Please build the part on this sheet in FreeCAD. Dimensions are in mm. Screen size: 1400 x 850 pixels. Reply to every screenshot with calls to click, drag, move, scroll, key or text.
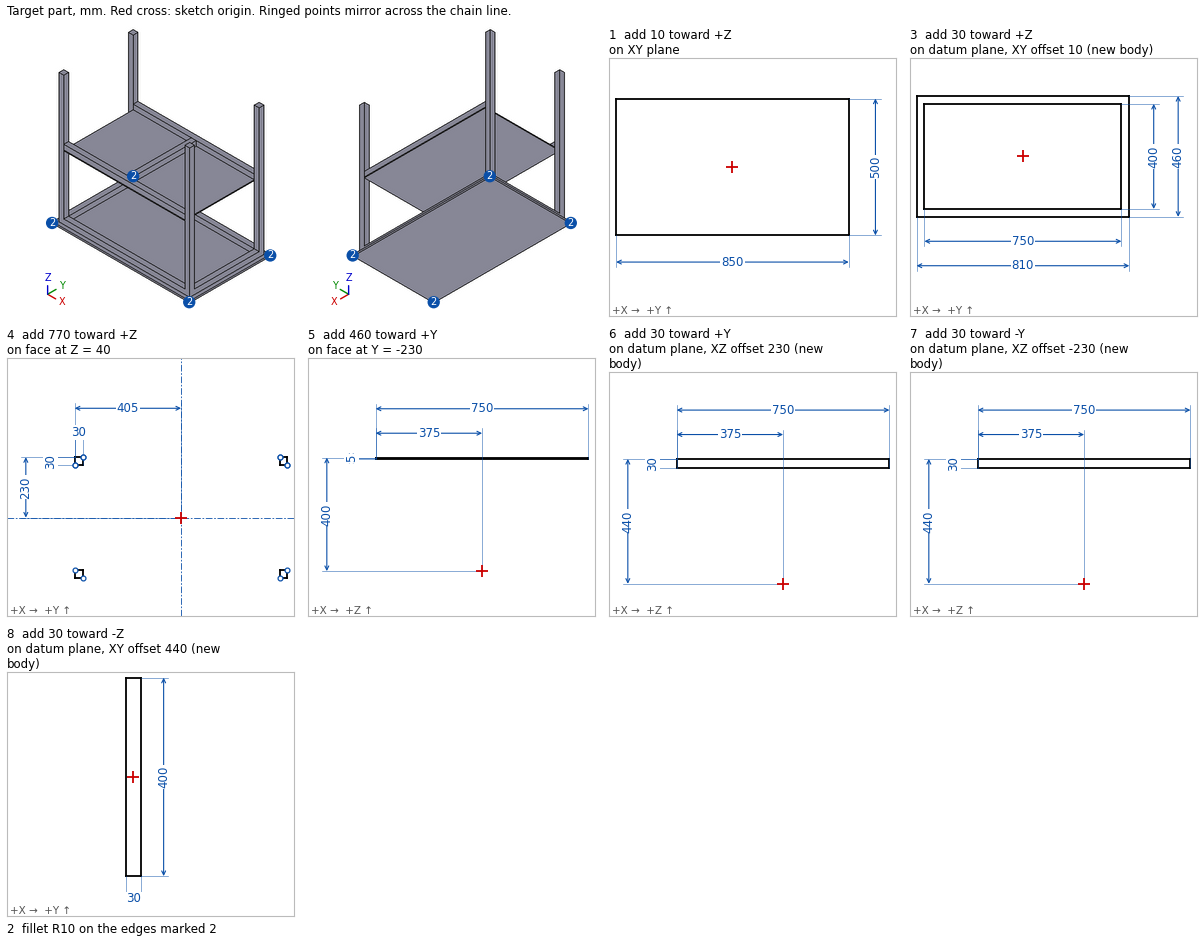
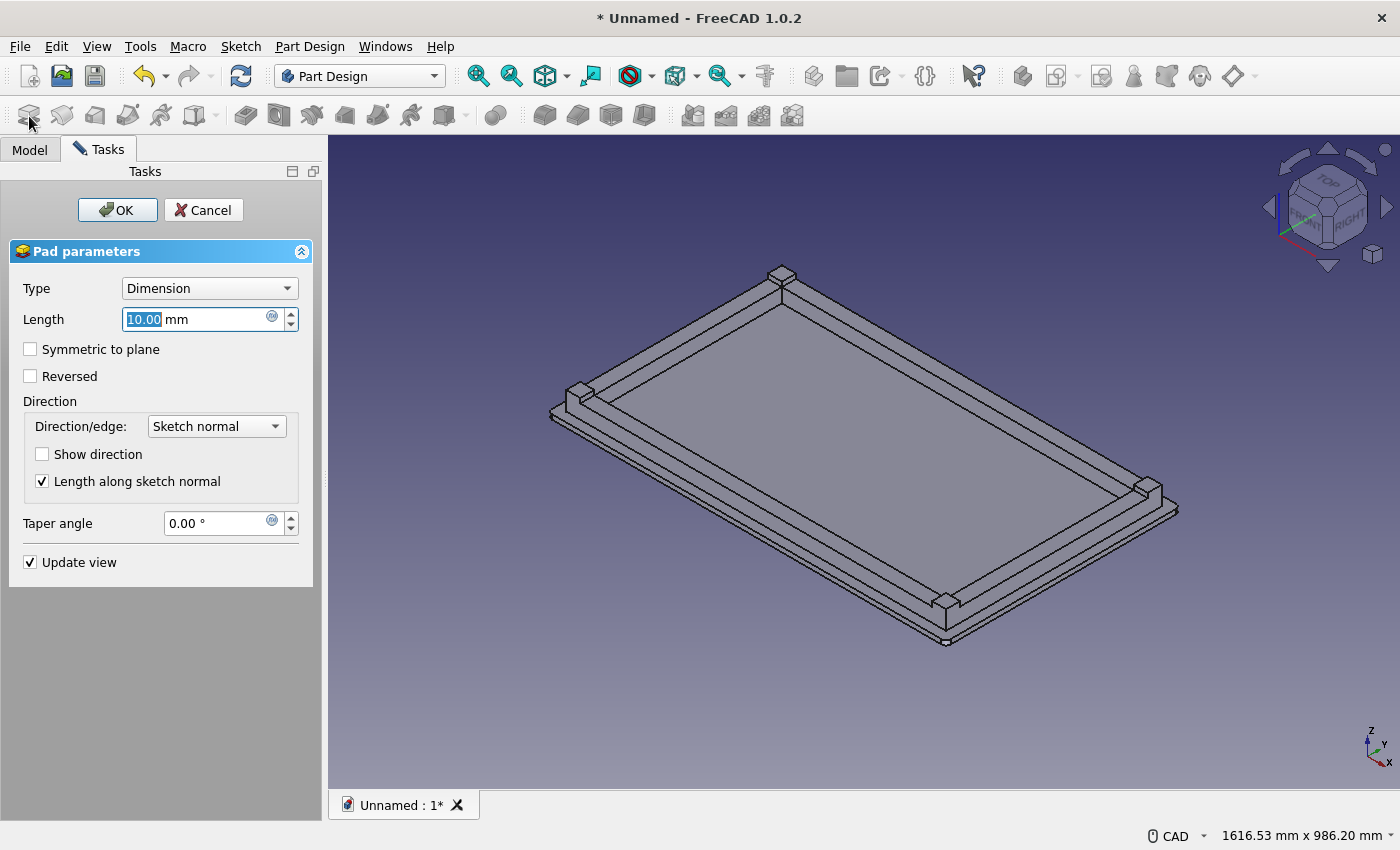
text(770)
key(Tab)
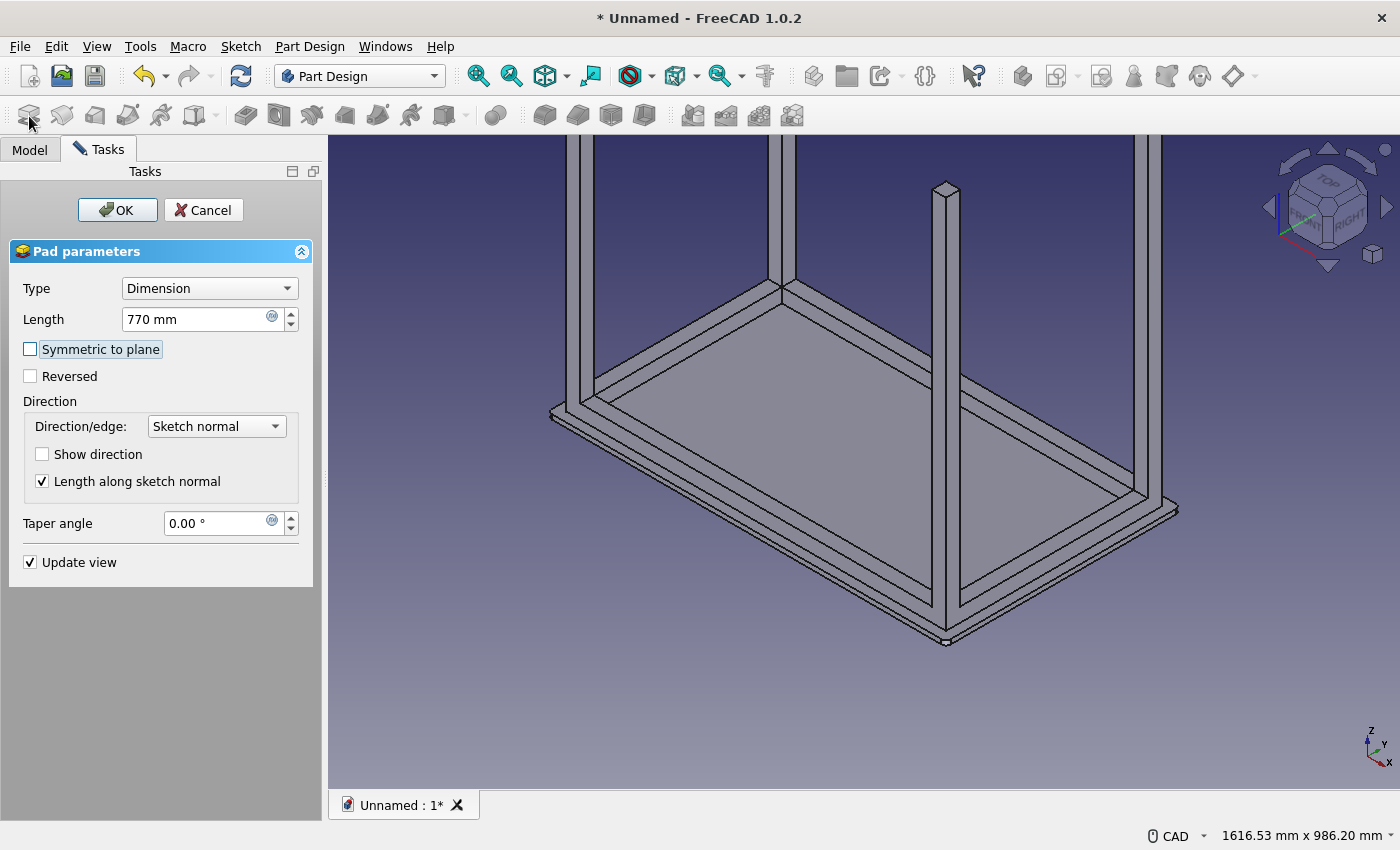
click(118, 210)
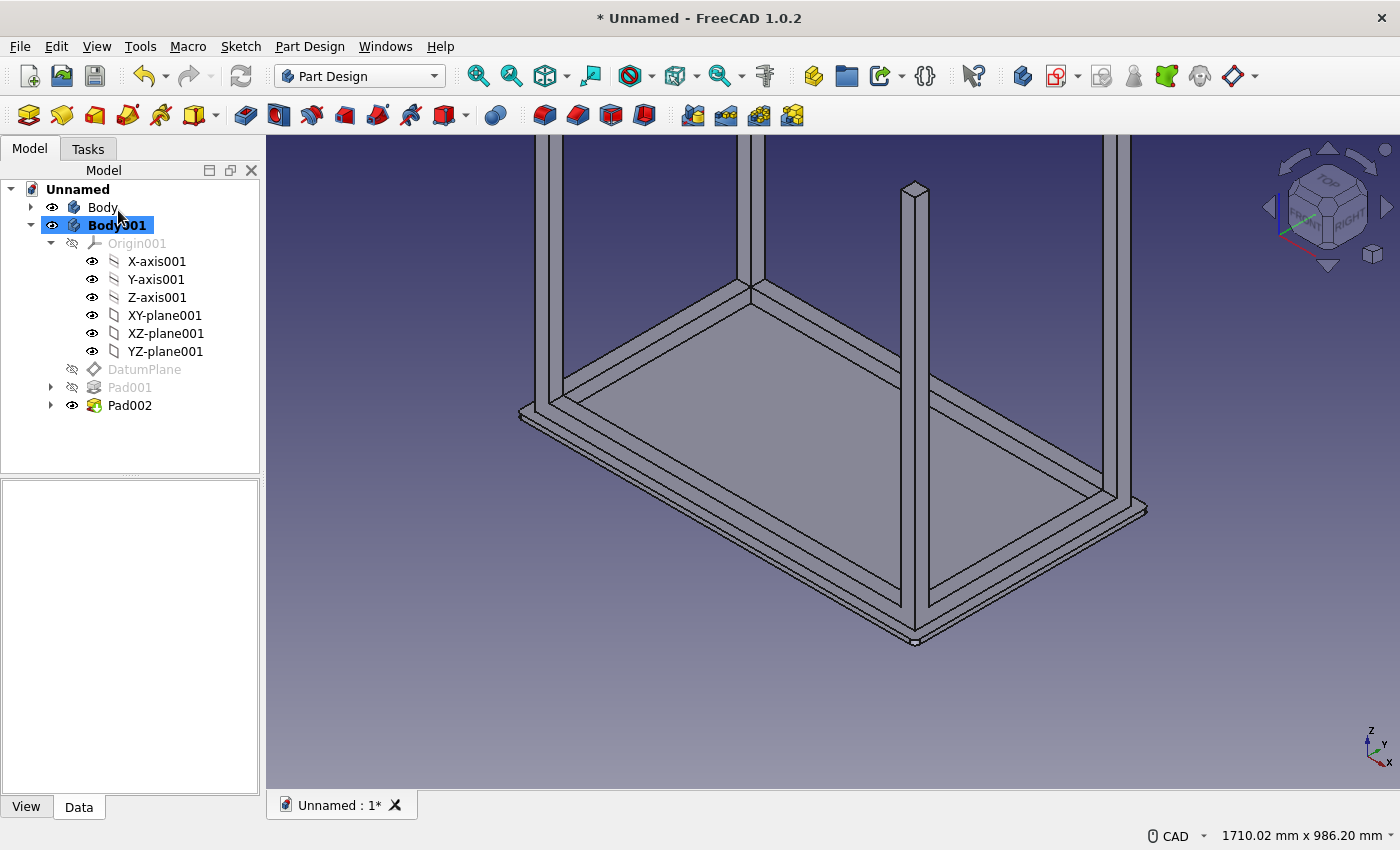
click(479, 76)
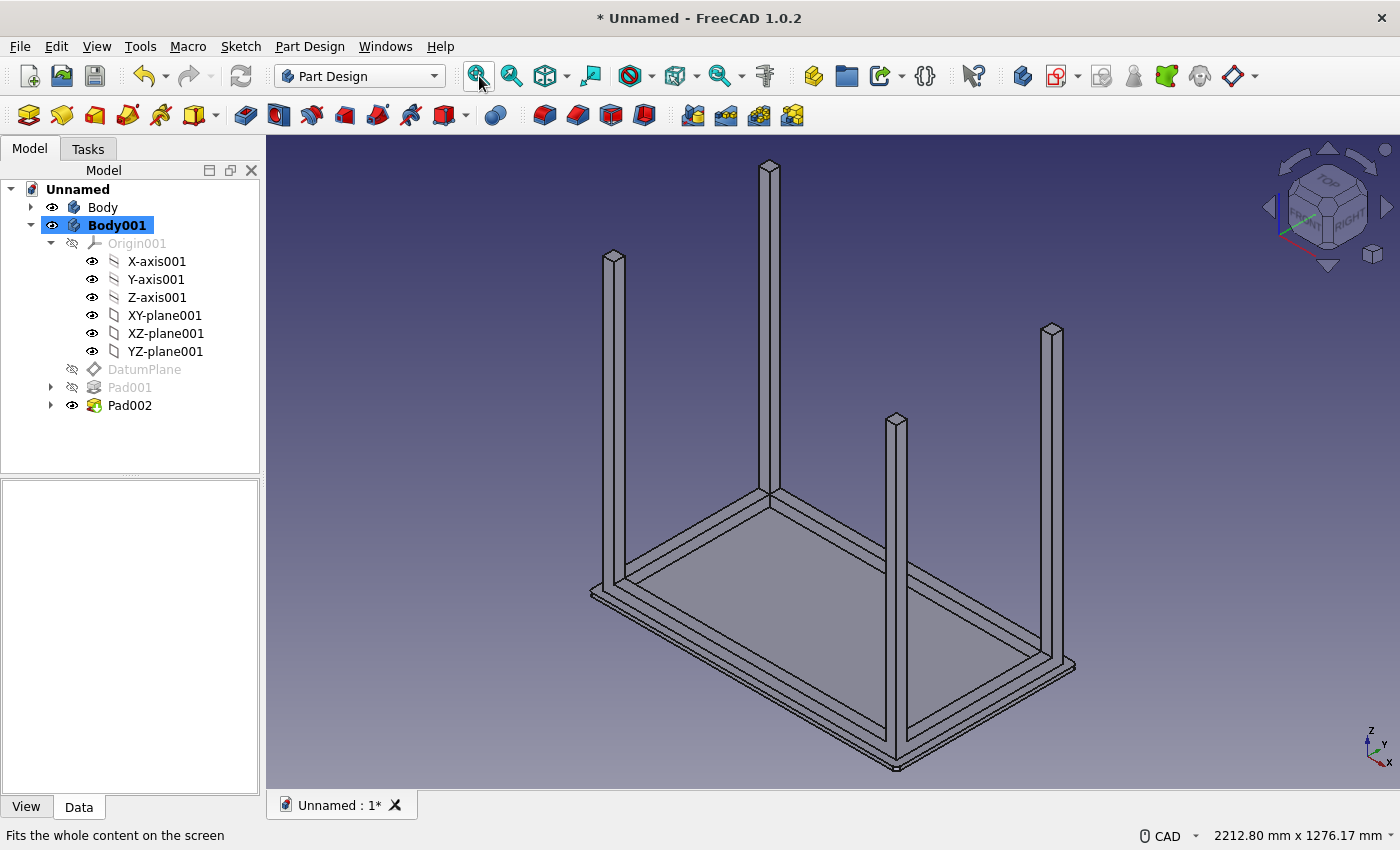
scroll(893, 641, up, 5)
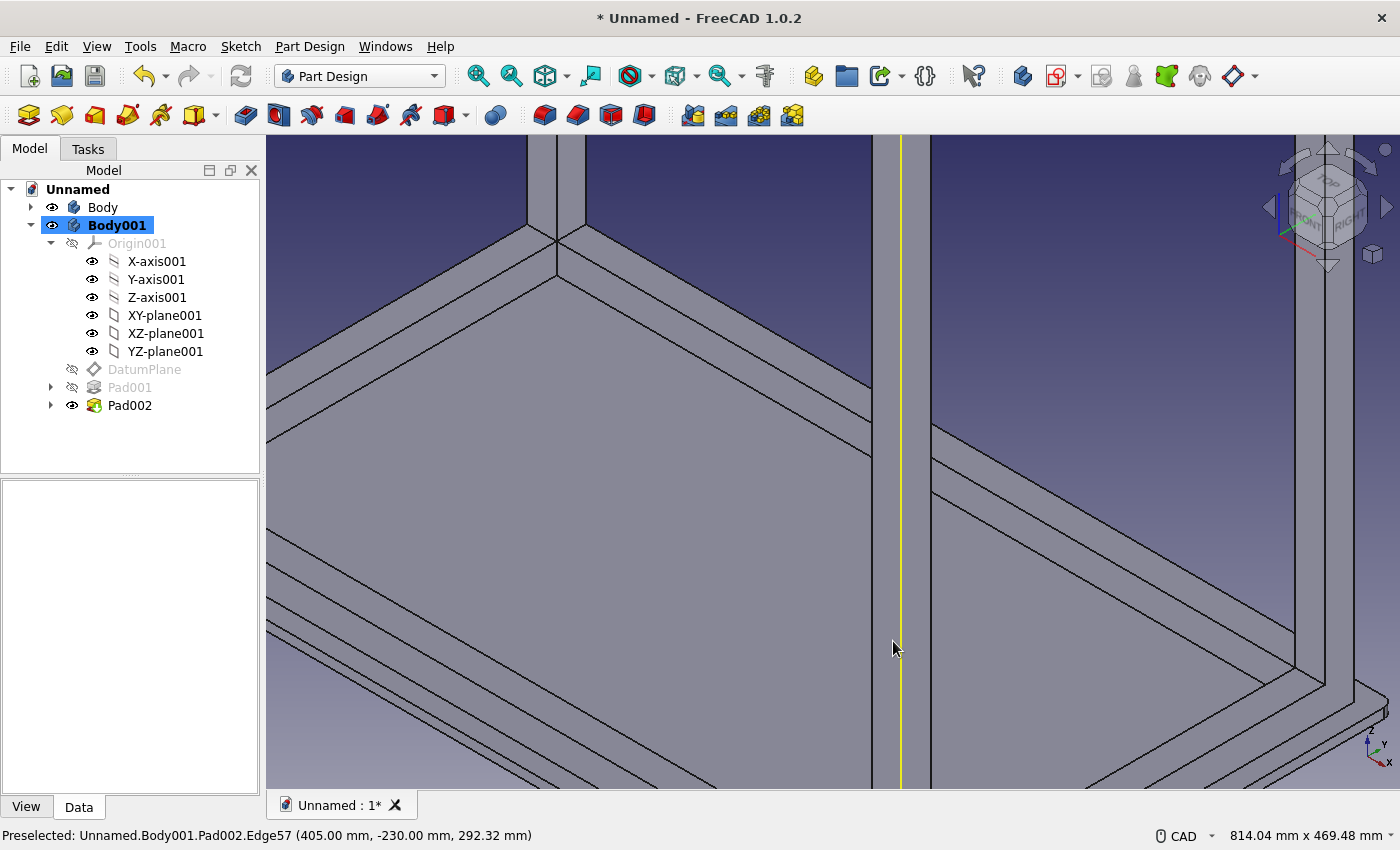
click(891, 642)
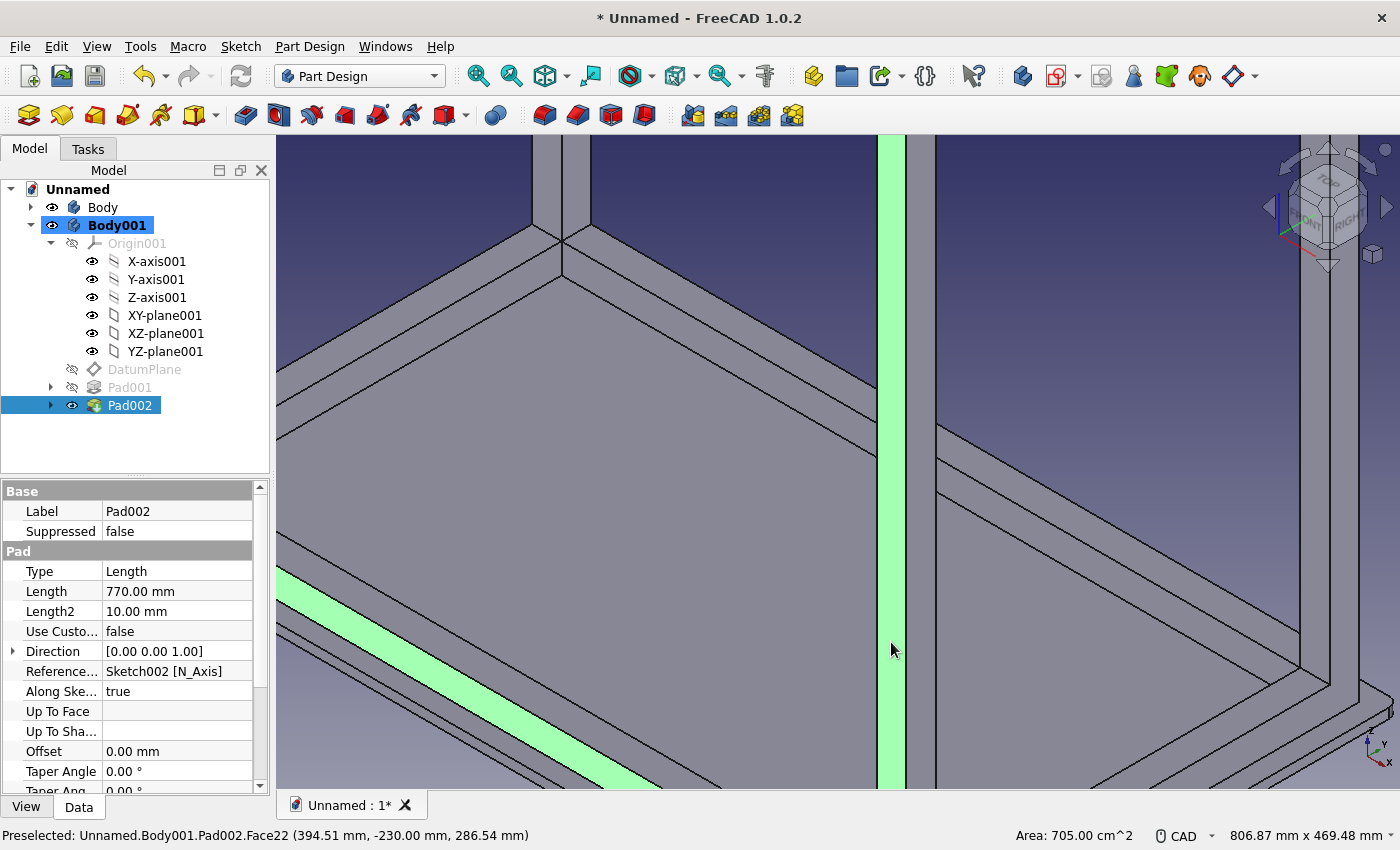
click(1056, 76)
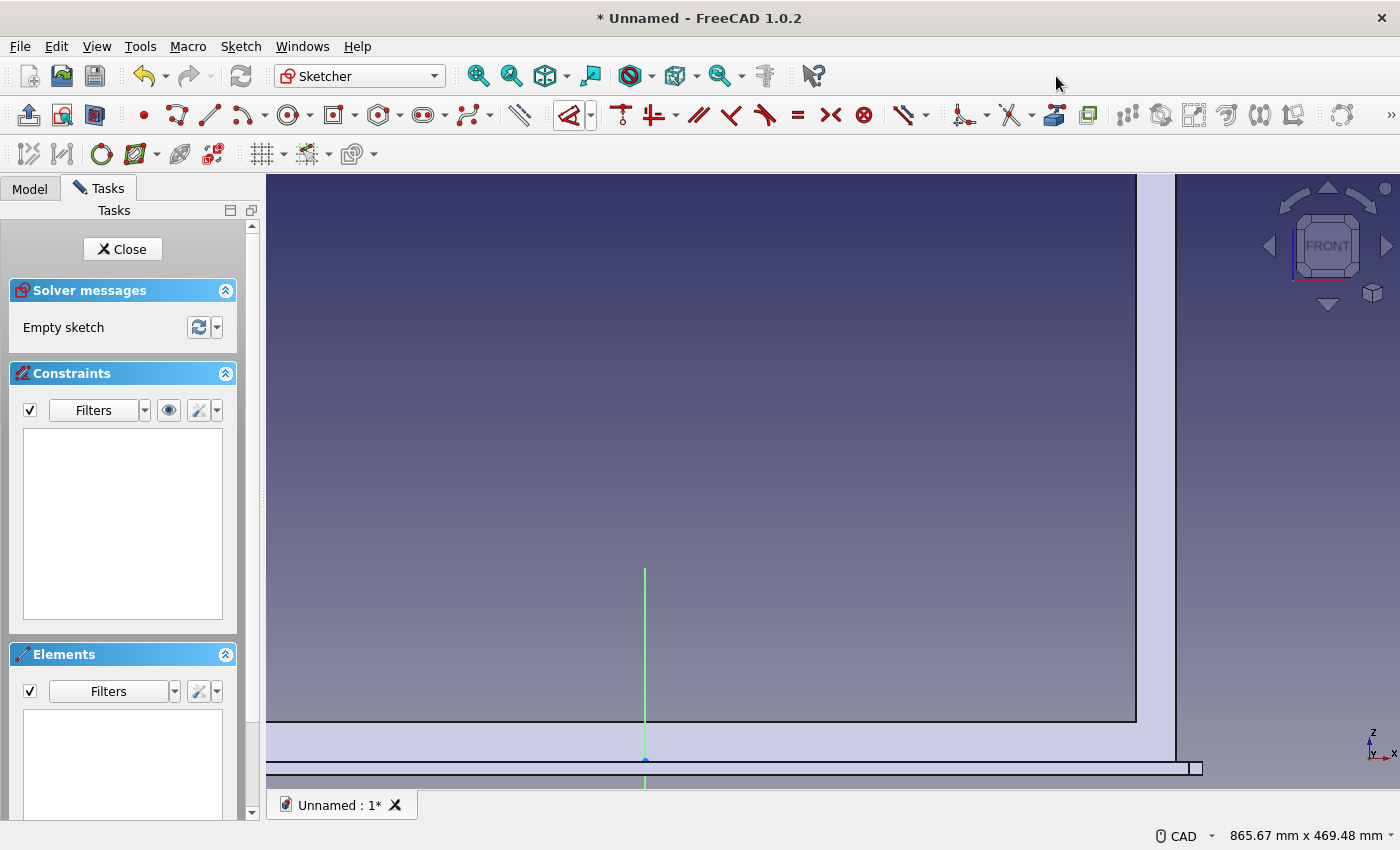
scroll(1007, 444, down, 2)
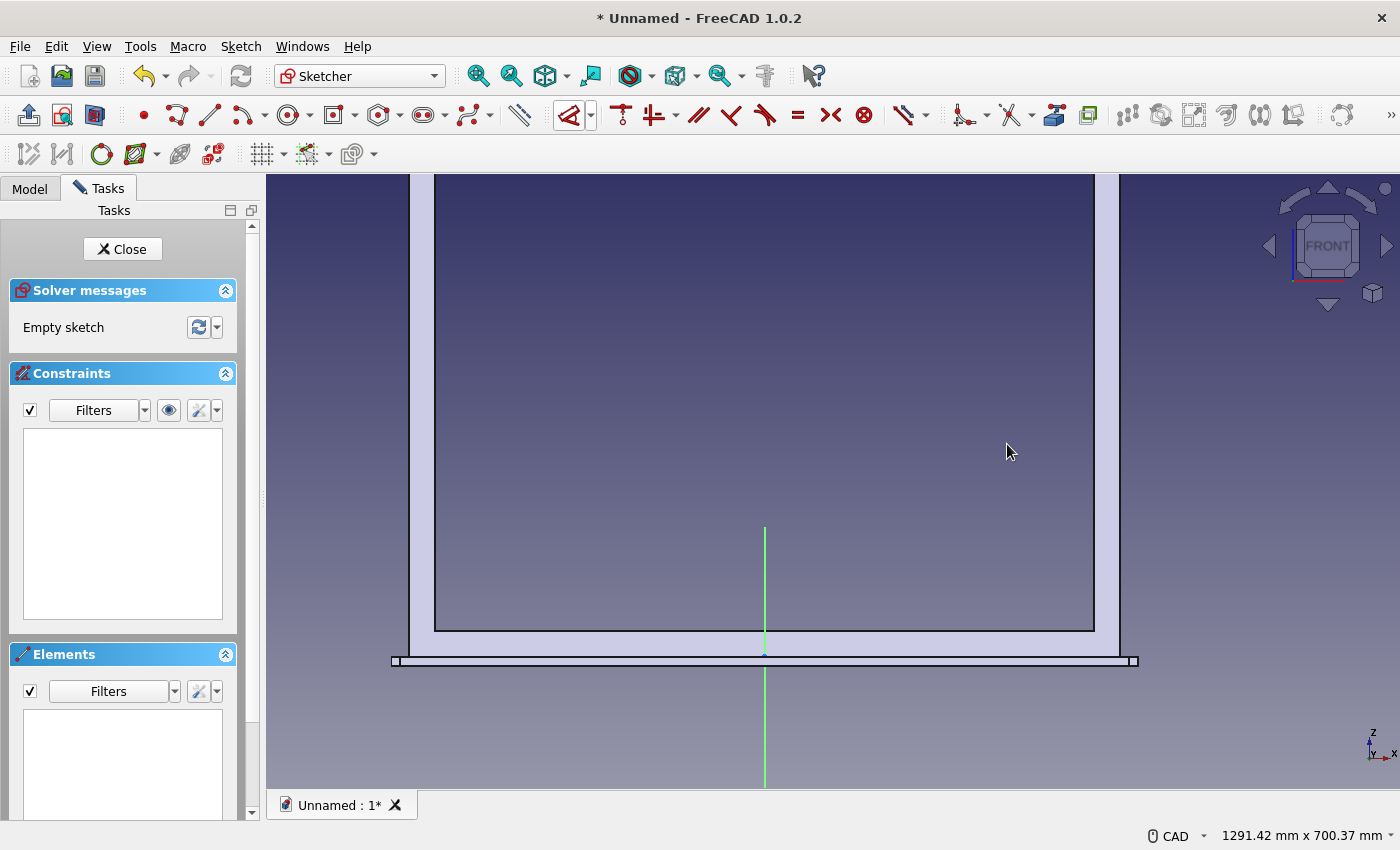
click(354, 116)